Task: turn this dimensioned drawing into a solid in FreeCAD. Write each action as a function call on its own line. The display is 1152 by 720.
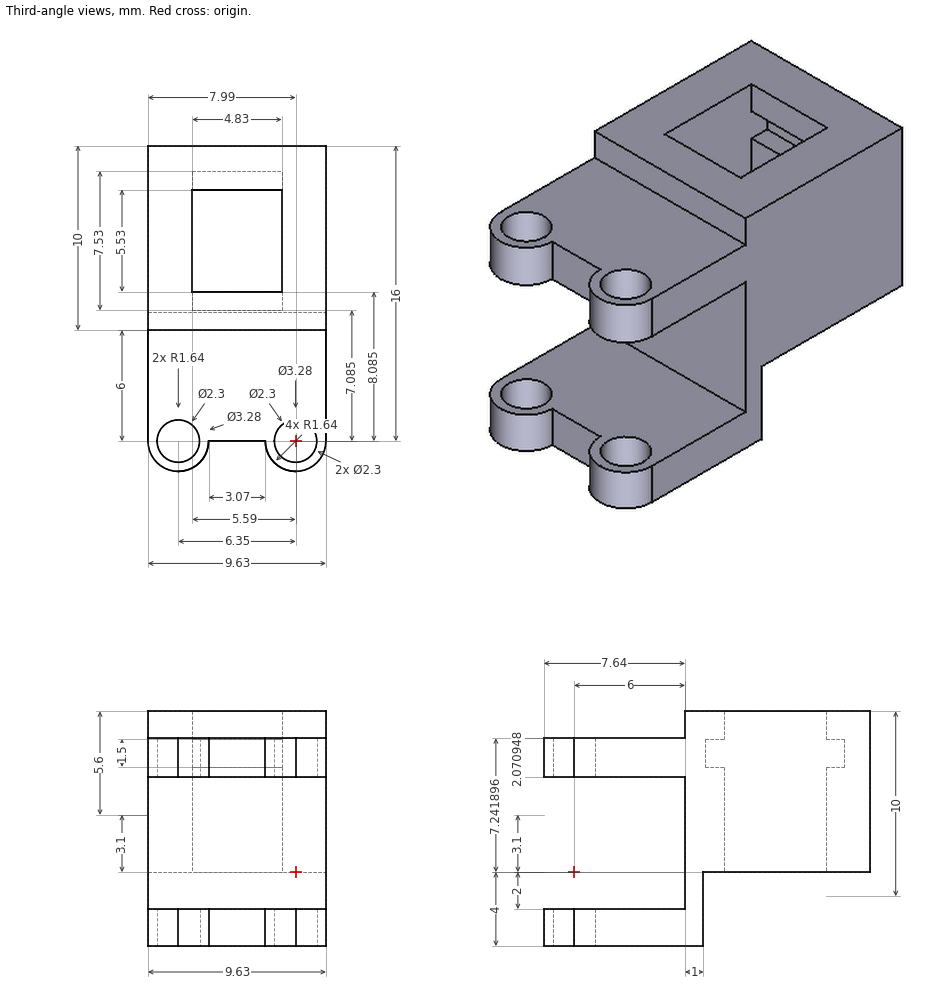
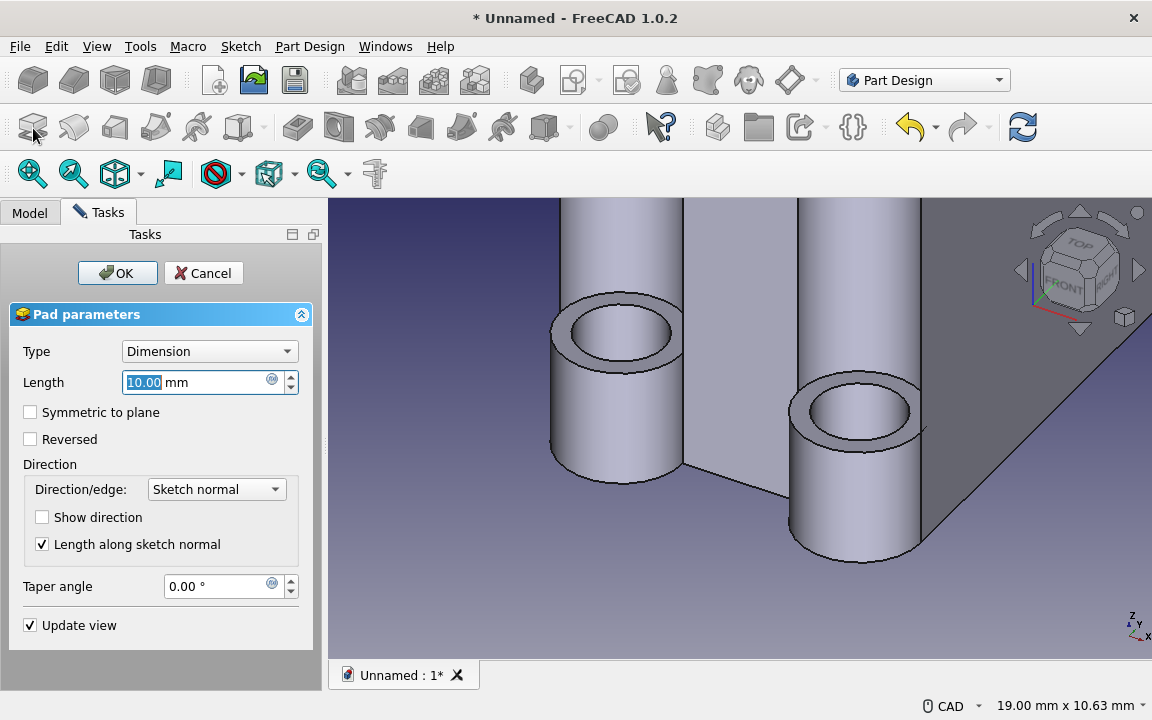
text(3.1)
key(Tab)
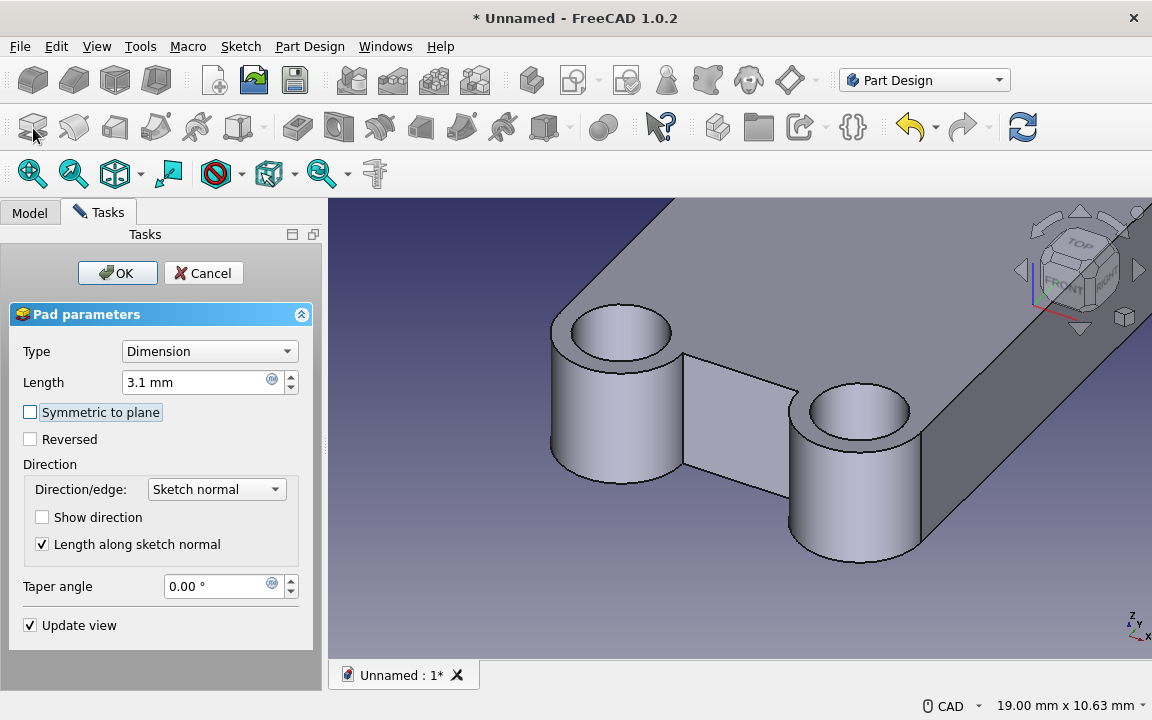
click(118, 273)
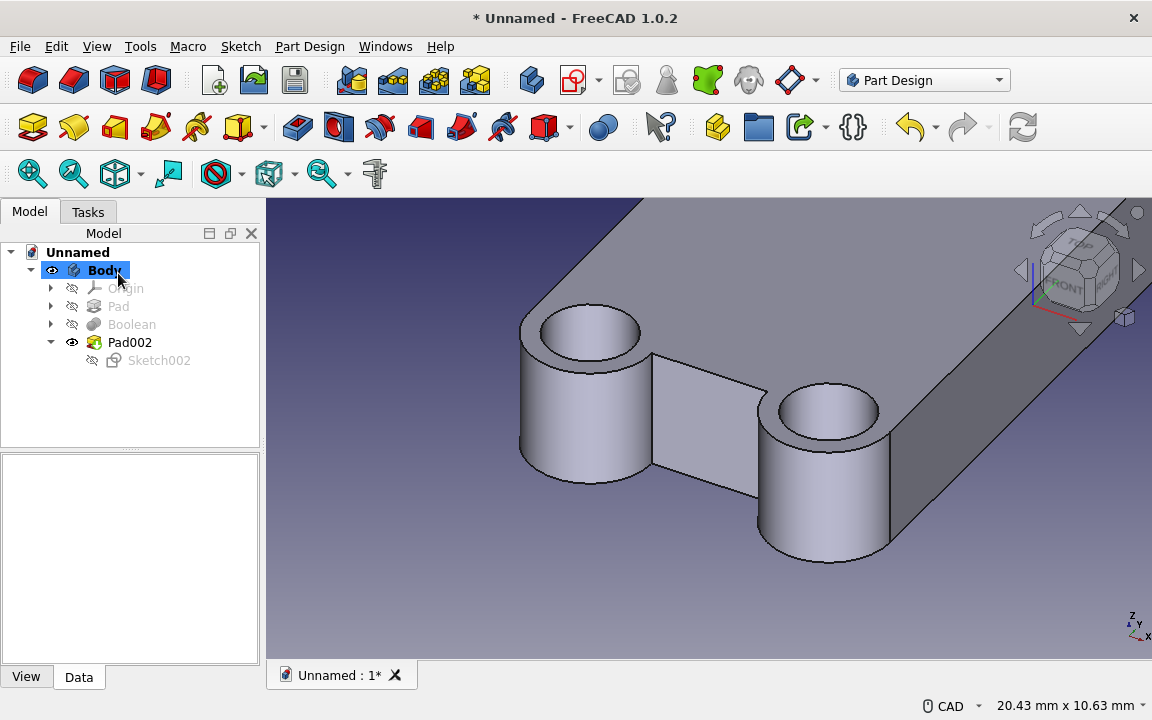
click(33, 174)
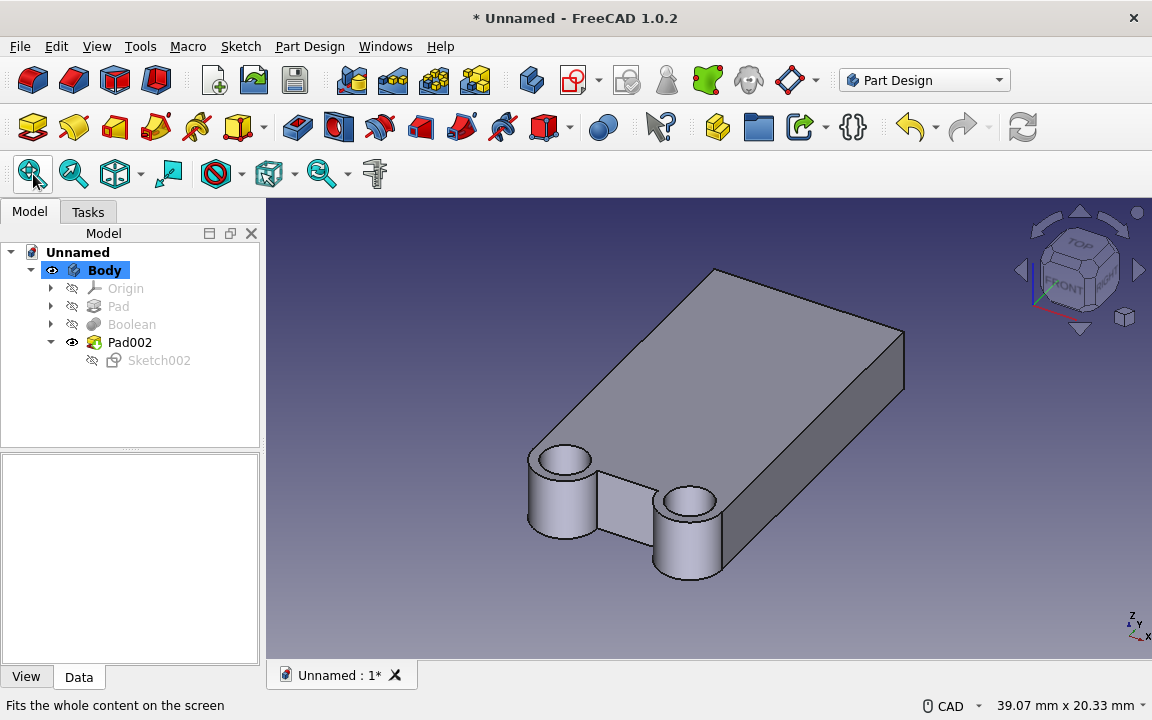
click(738, 370)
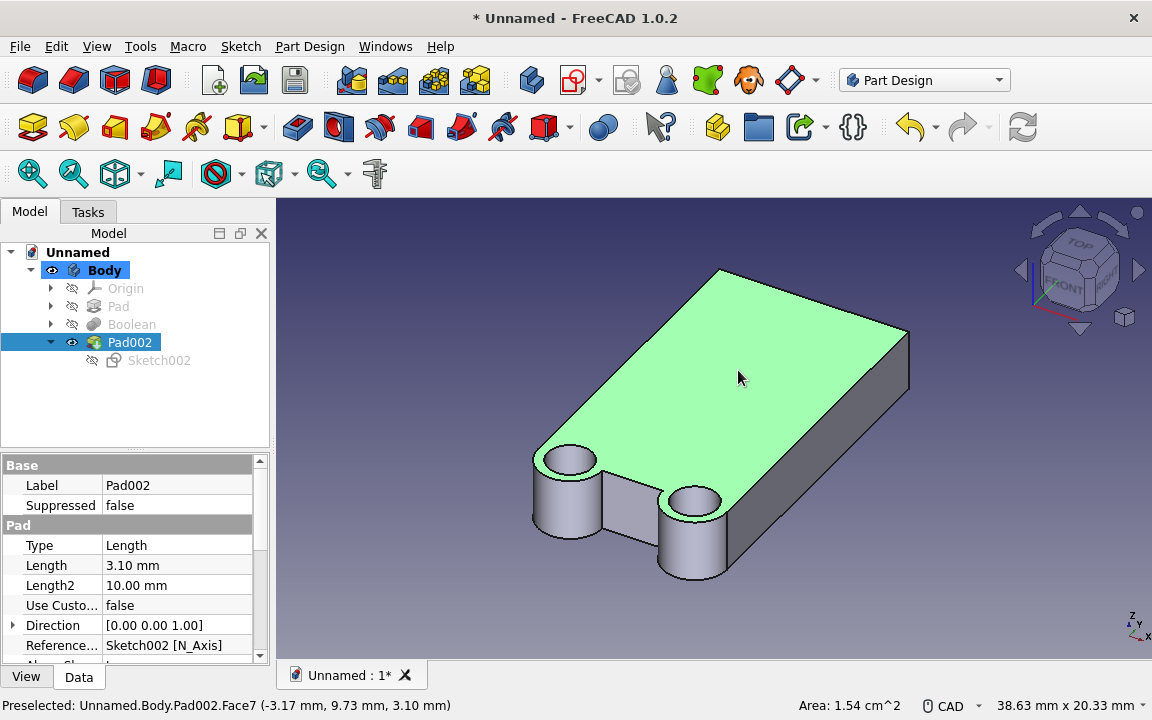
click(572, 80)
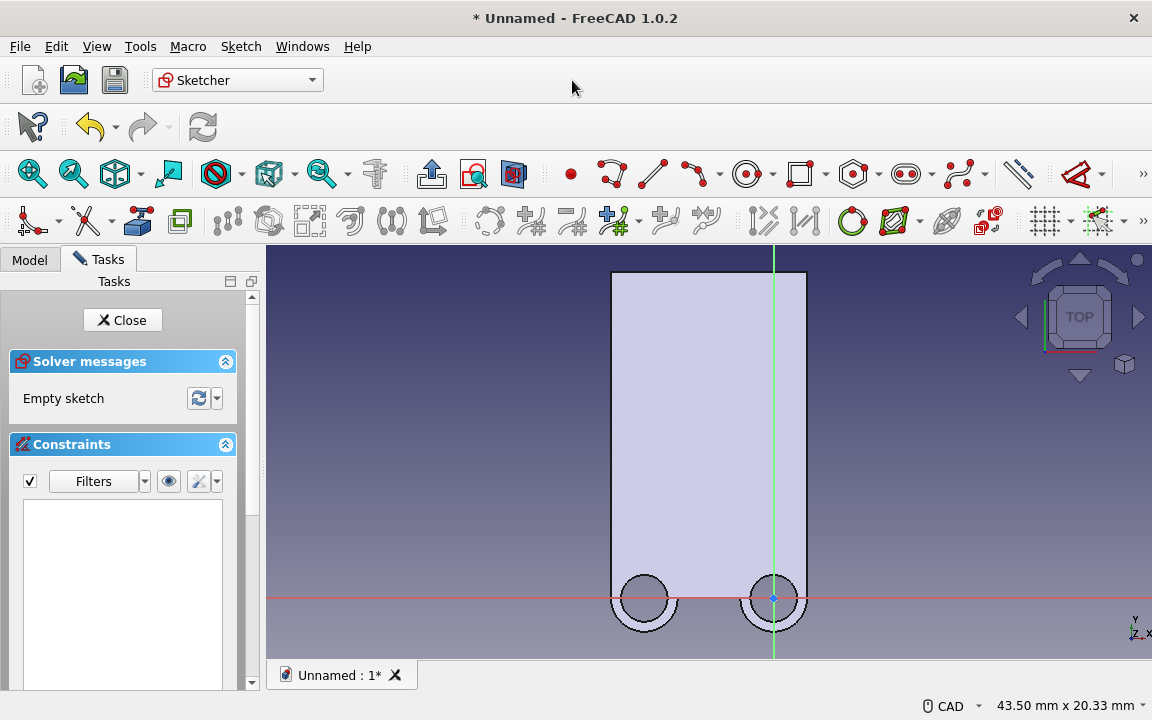
scroll(331, 527, down, 1)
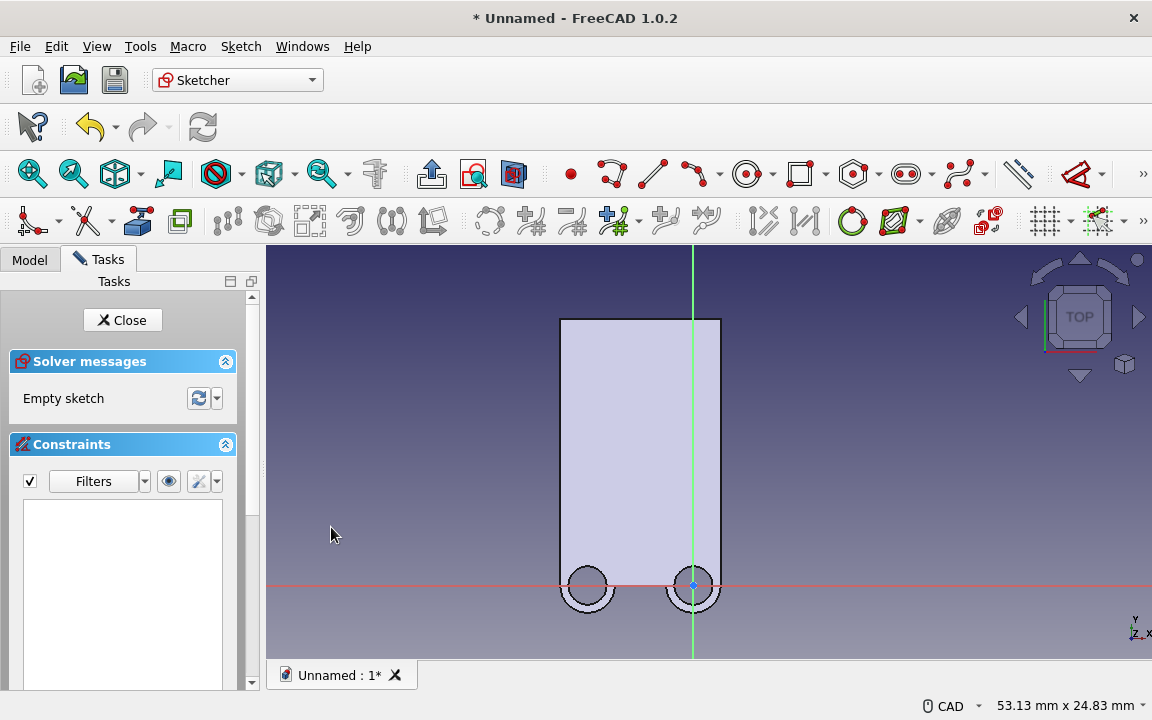
click(800, 174)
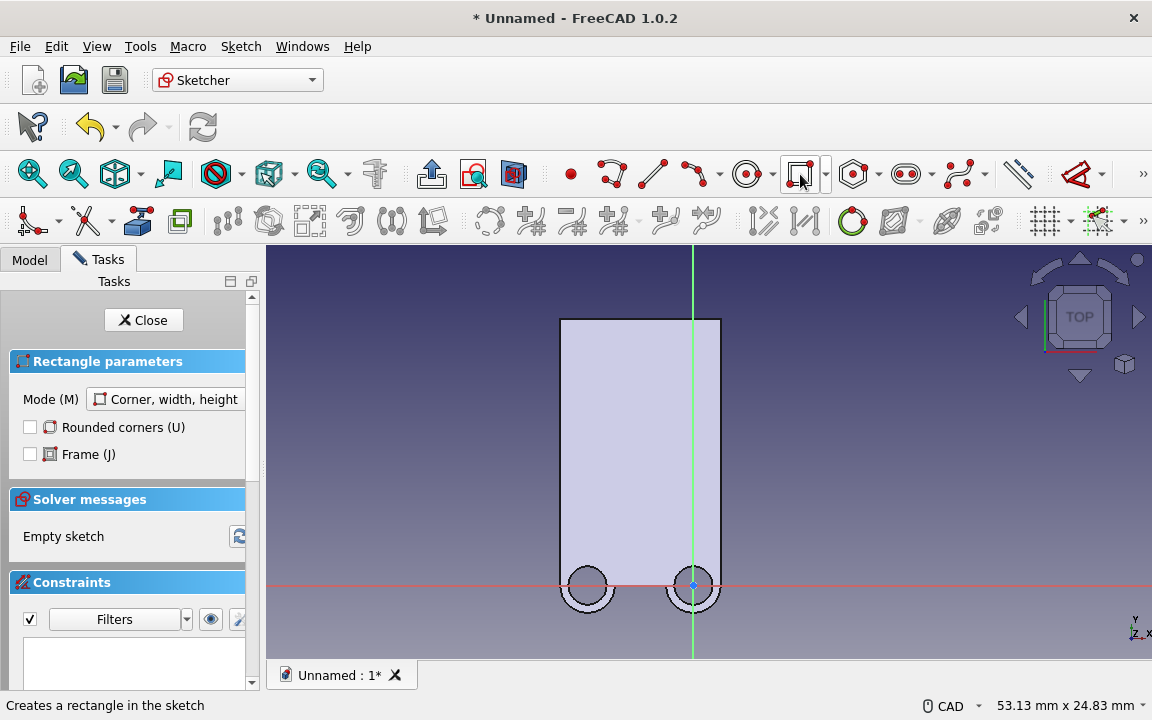
click(560, 319)
click(721, 485)
key(Escape)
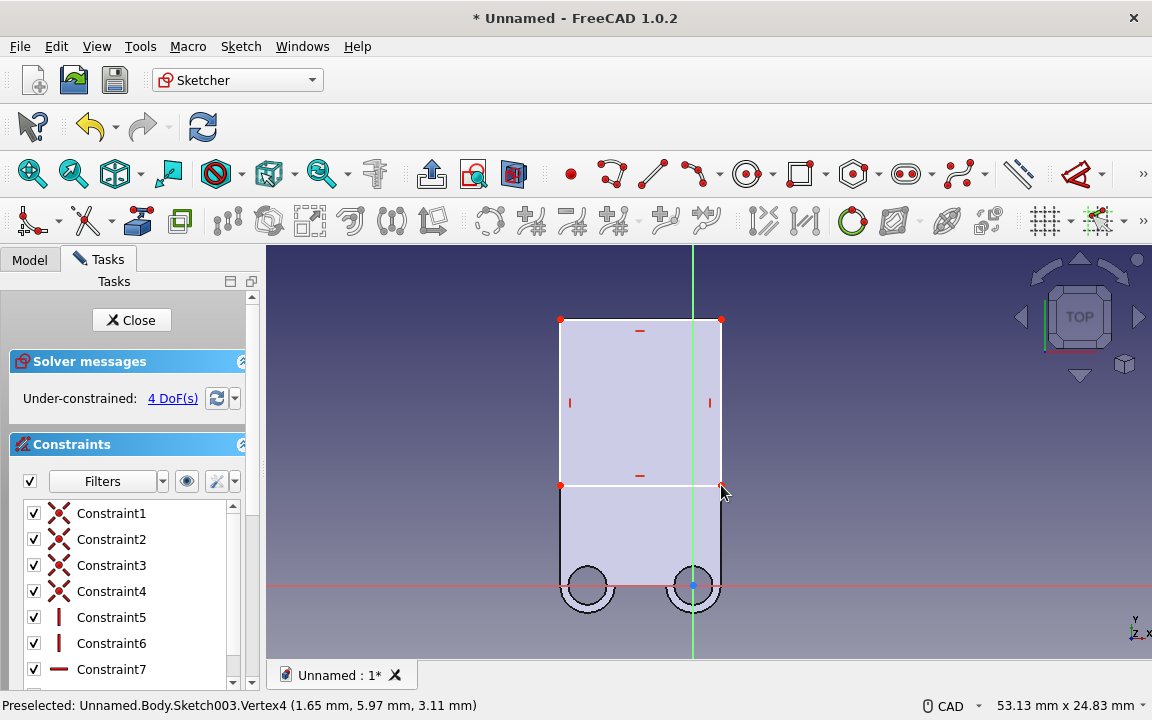
click(1076, 174)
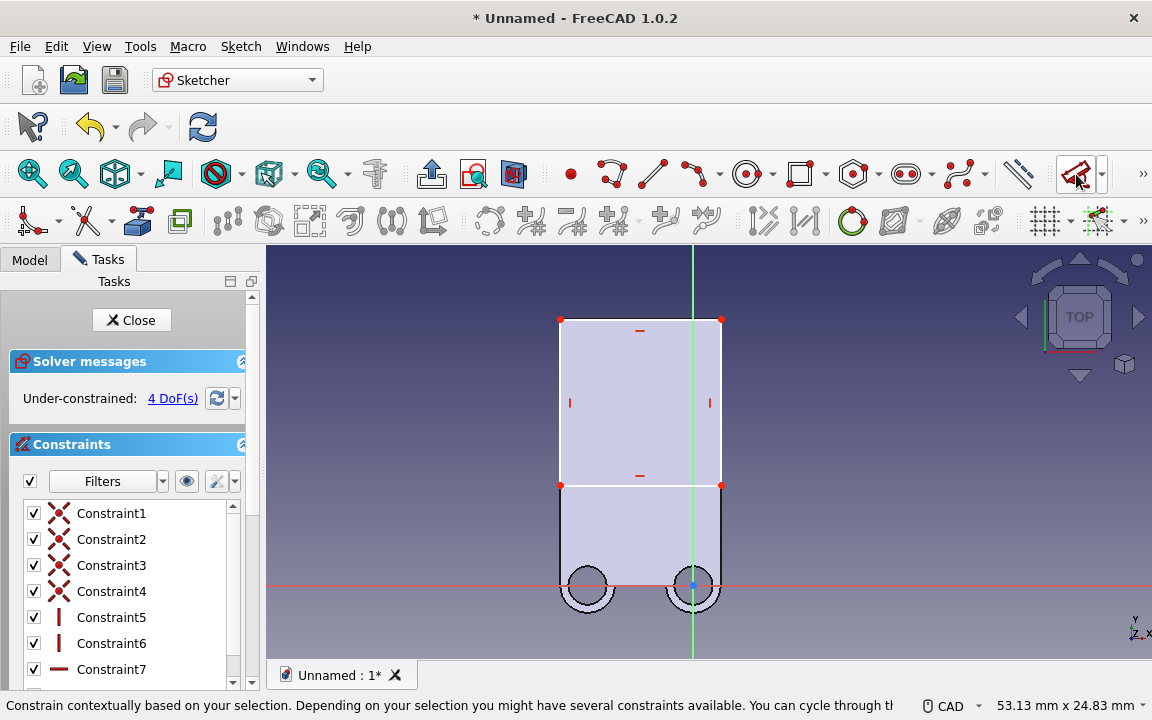
click(560, 370)
click(526, 403)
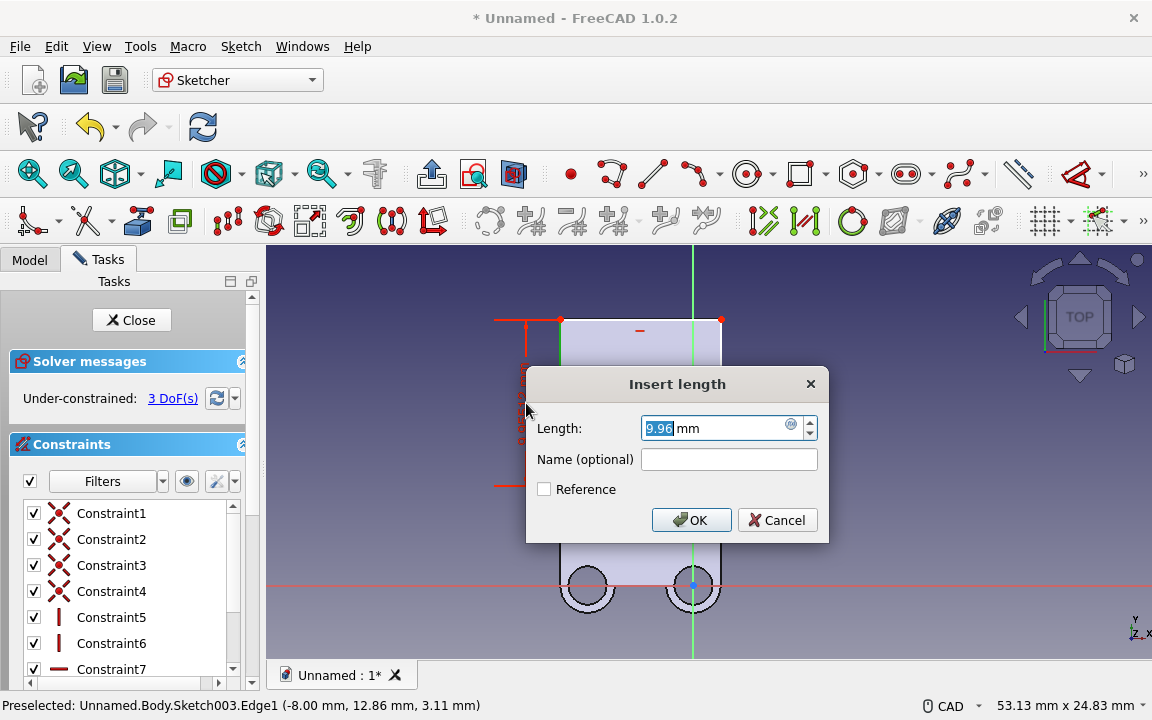
text(10)
key(Return)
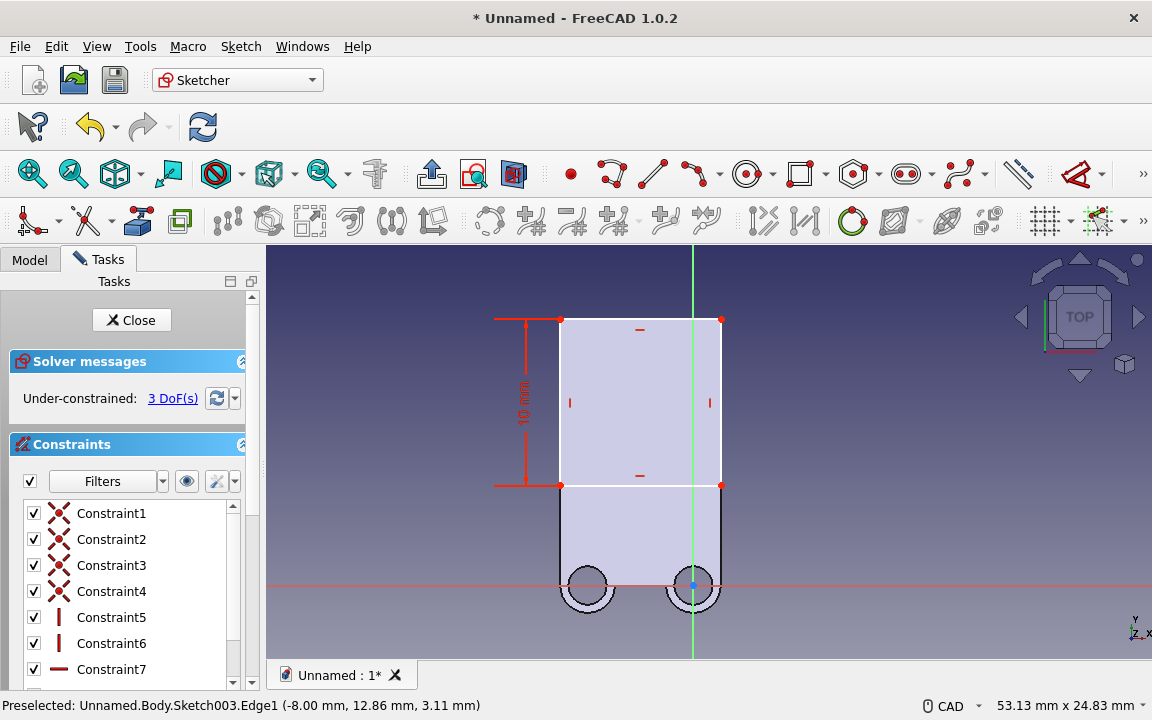
click(560, 486)
click(526, 536)